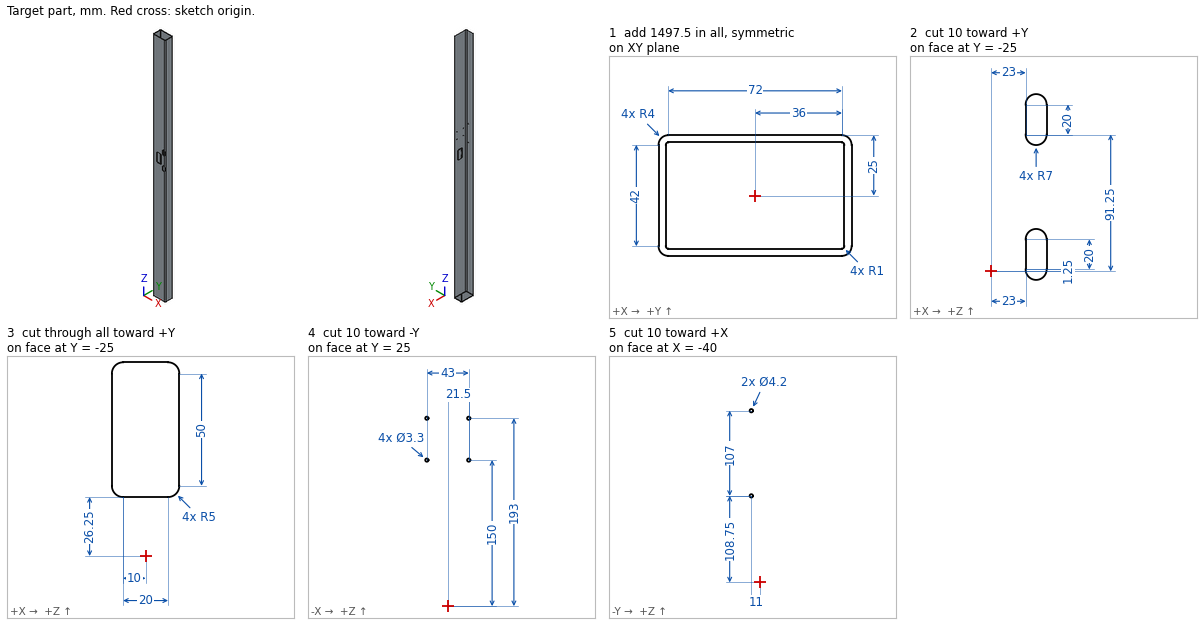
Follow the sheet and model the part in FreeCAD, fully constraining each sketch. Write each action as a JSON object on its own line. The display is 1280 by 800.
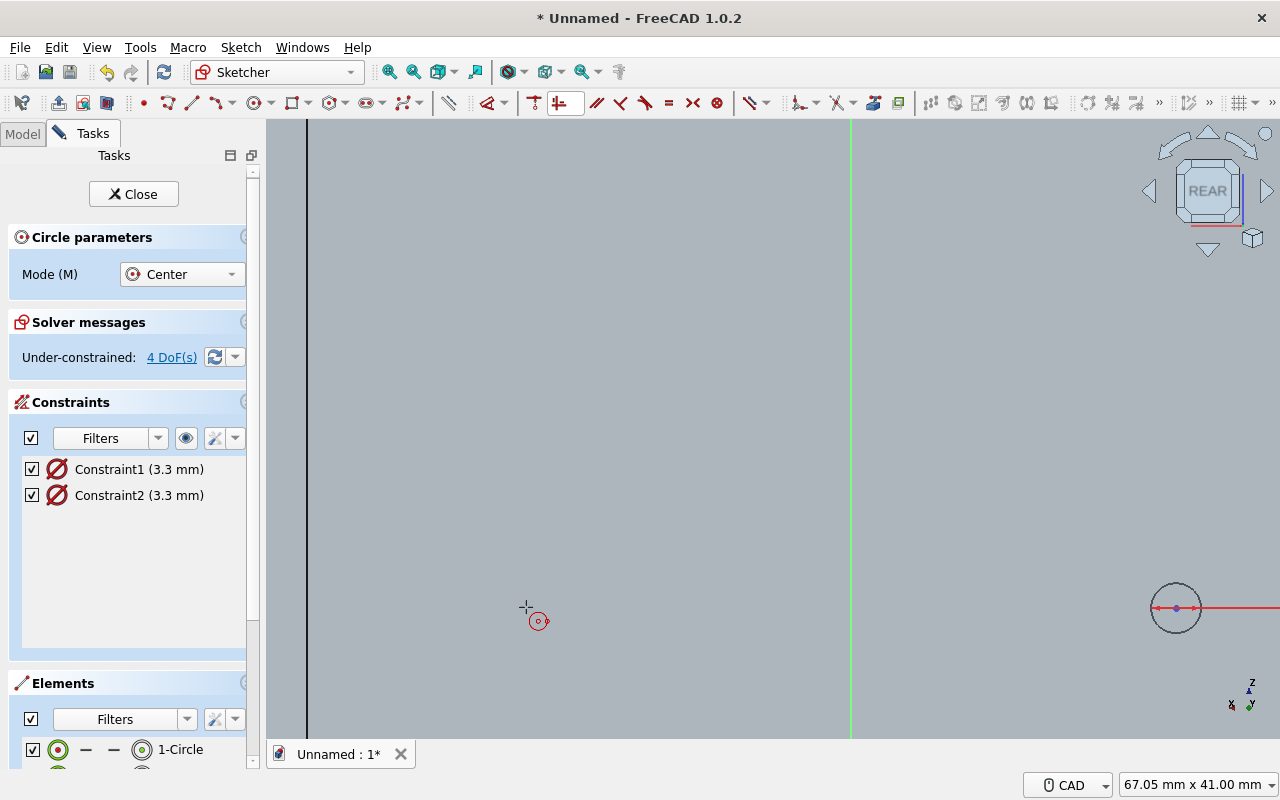
{"action": "left_click", "coordinate": [526, 607]}
{"action": "mouse_move", "coordinate": [544, 589]}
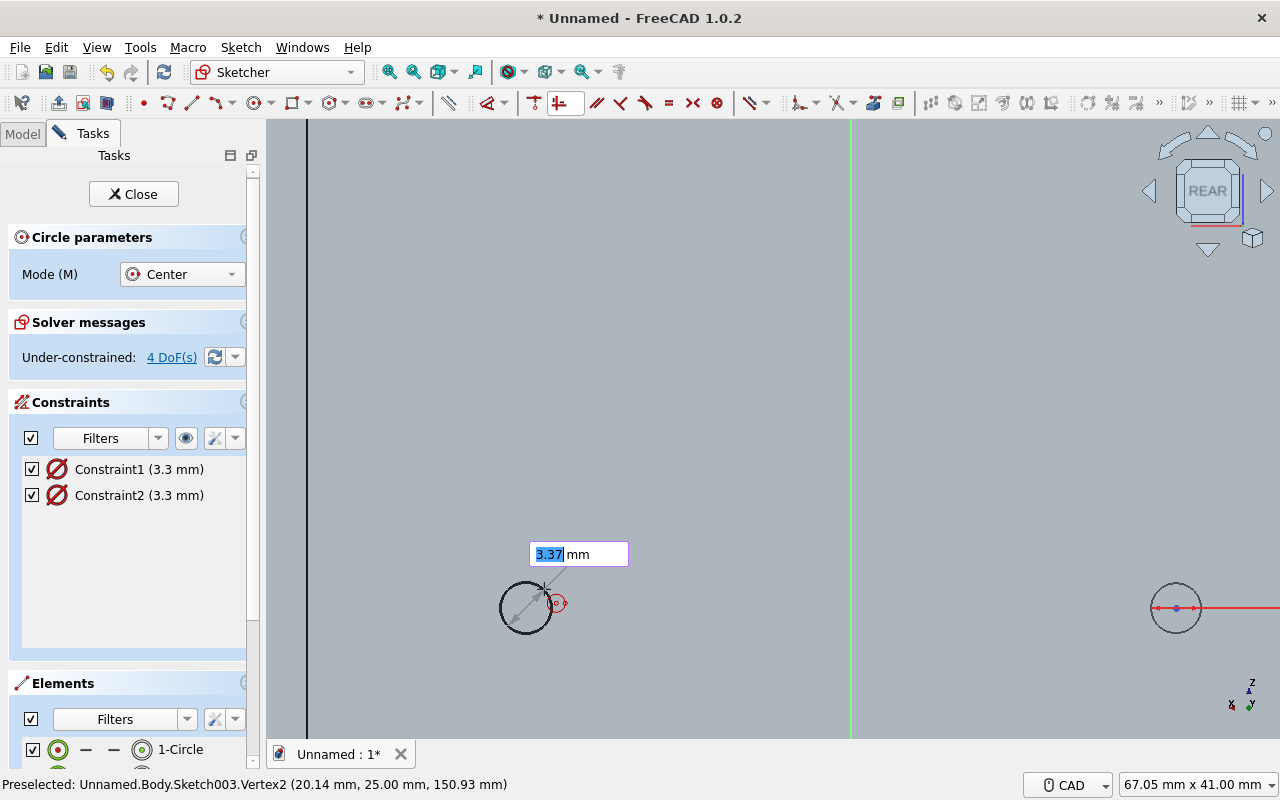
{"action": "type", "text": "3.3"}
{"action": "key", "text": "Return"}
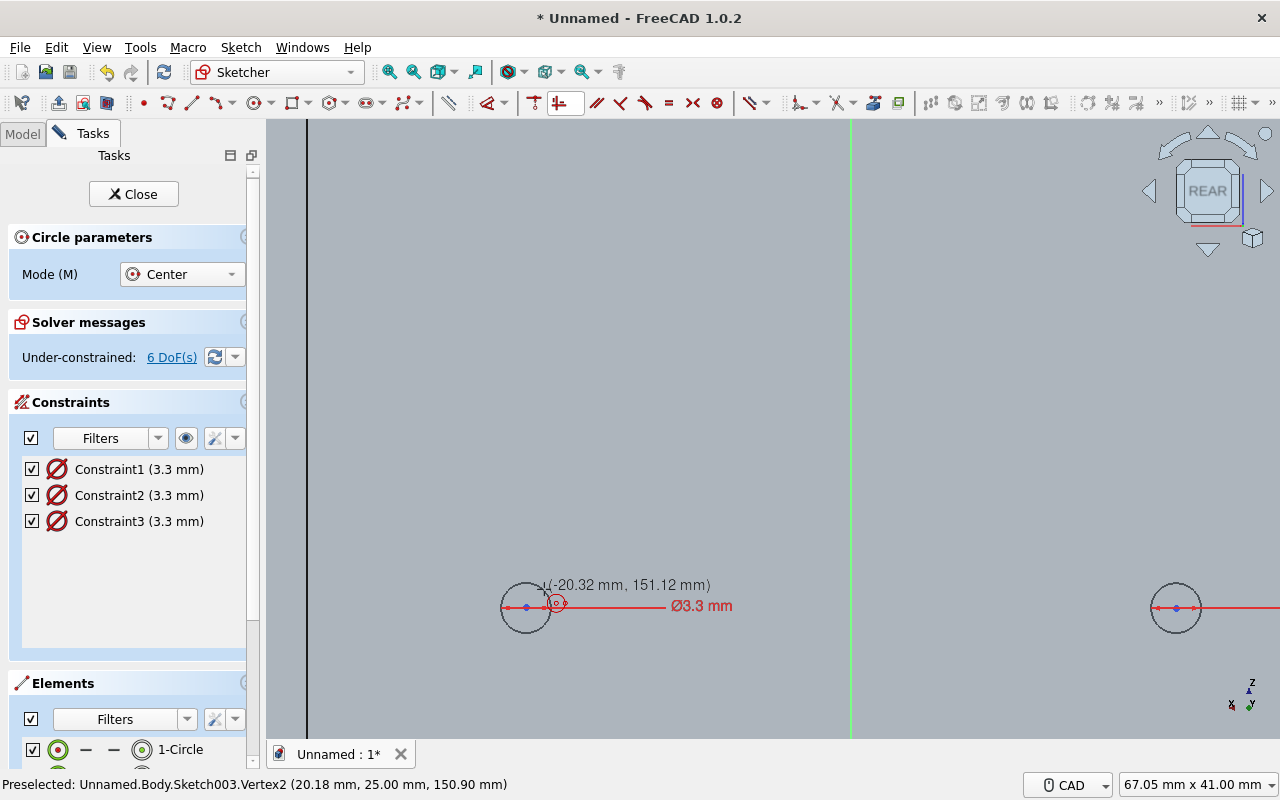
{"action": "scroll", "coordinate": [526, 608], "scroll_direction": "down", "scroll_amount": 3}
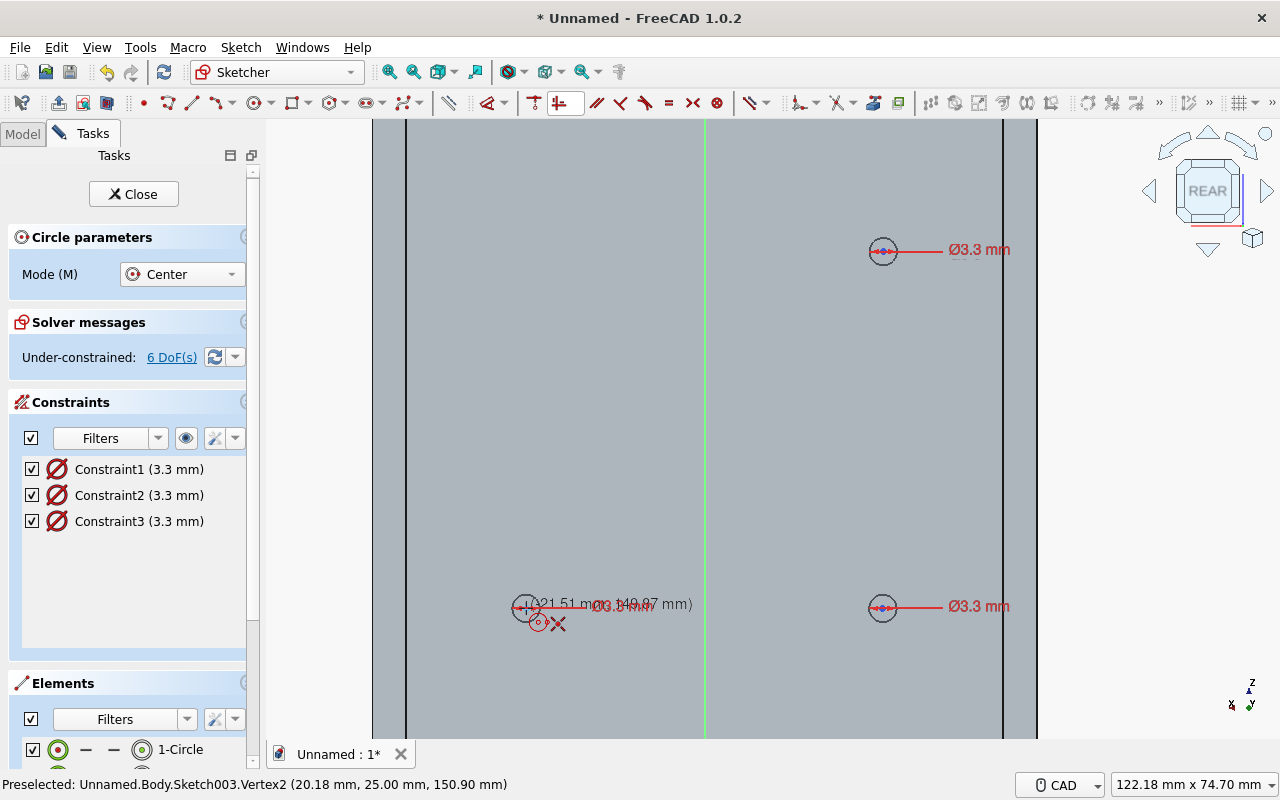
{"action": "scroll", "coordinate": [526, 251], "scroll_direction": "up", "scroll_amount": 3}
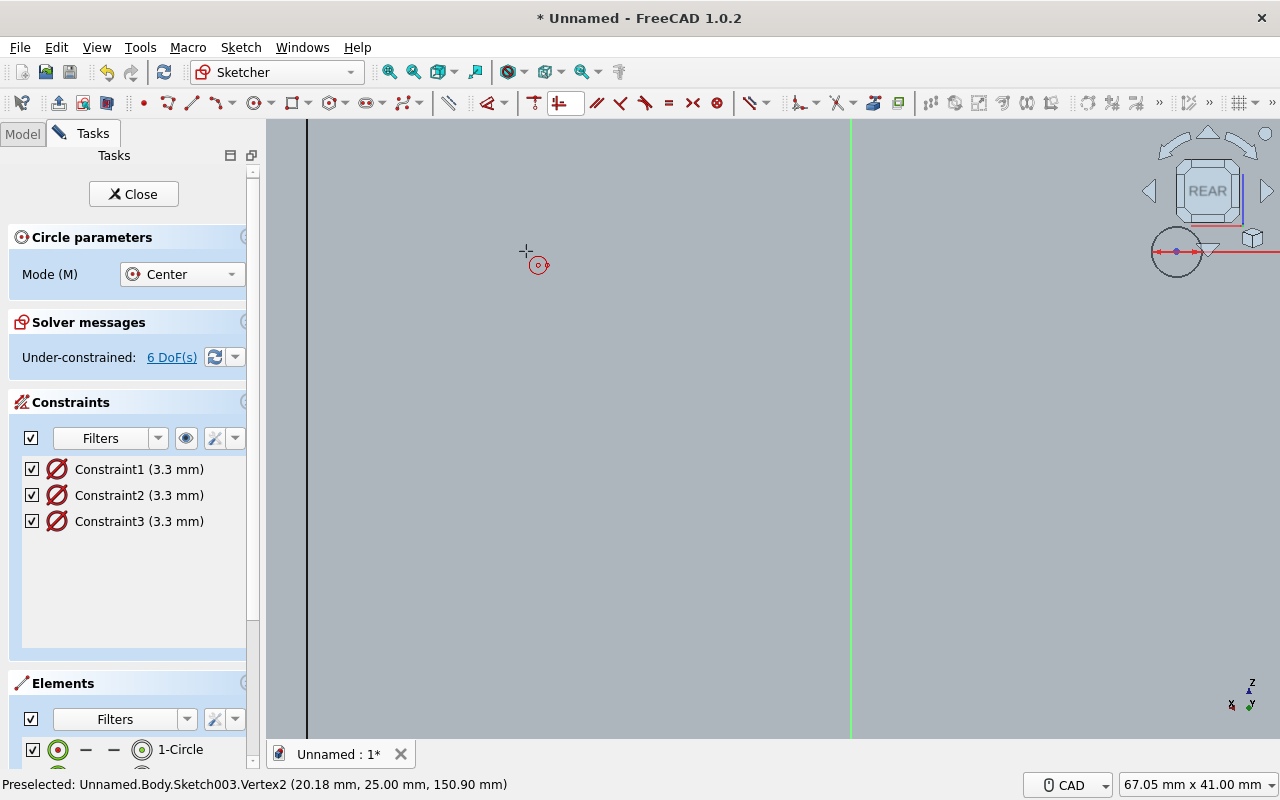
{"action": "left_click", "coordinate": [526, 251]}
{"action": "mouse_move", "coordinate": [544, 233]}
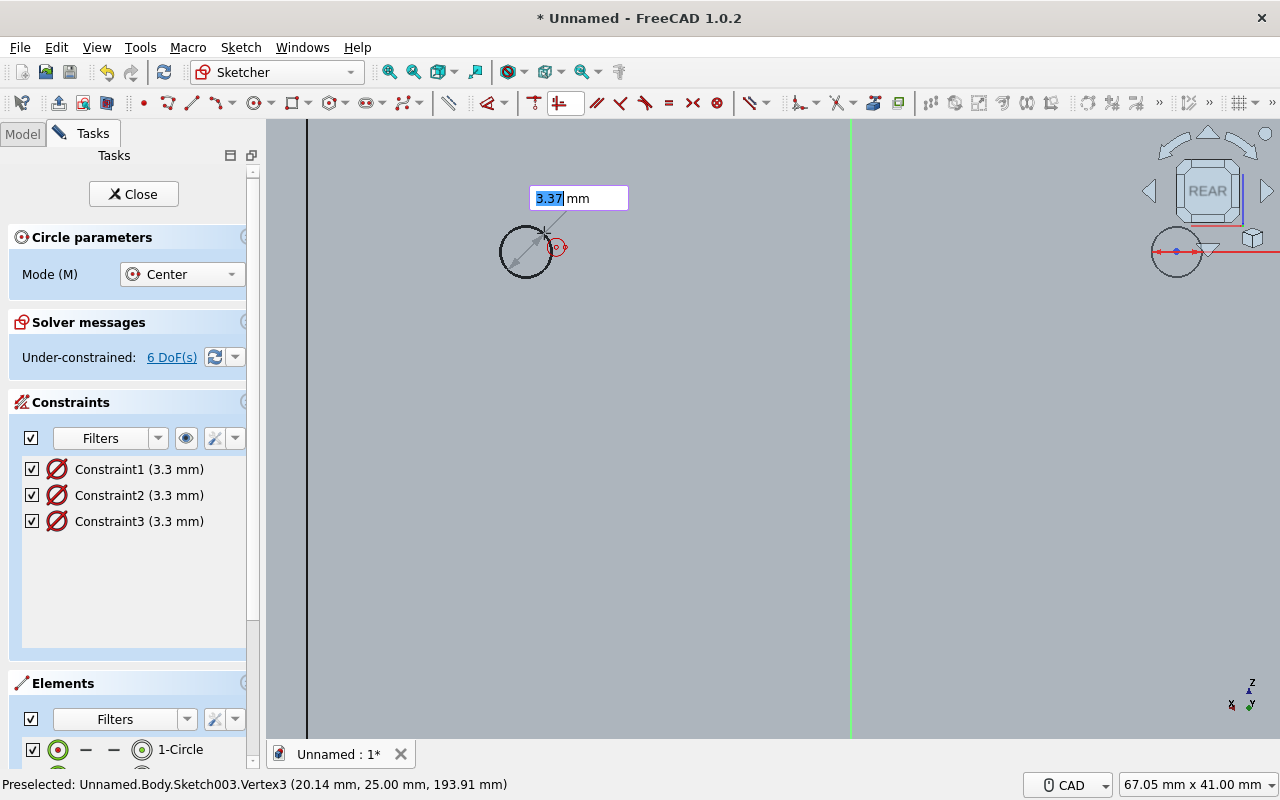
{"action": "type", "text": "3.3"}
{"action": "key", "text": "Return"}
{"action": "key", "text": "Escape"}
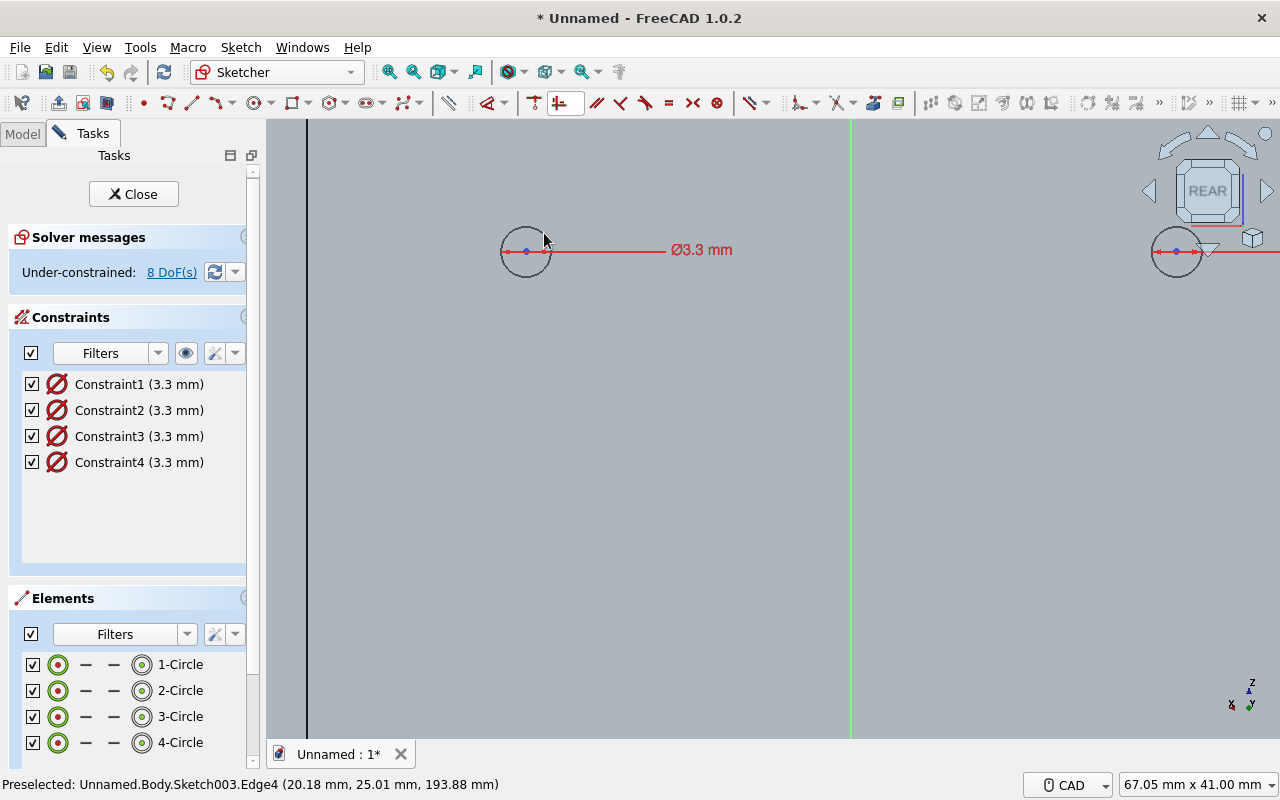
{"action": "scroll", "coordinate": [526, 250], "scroll_direction": "down", "scroll_amount": 3}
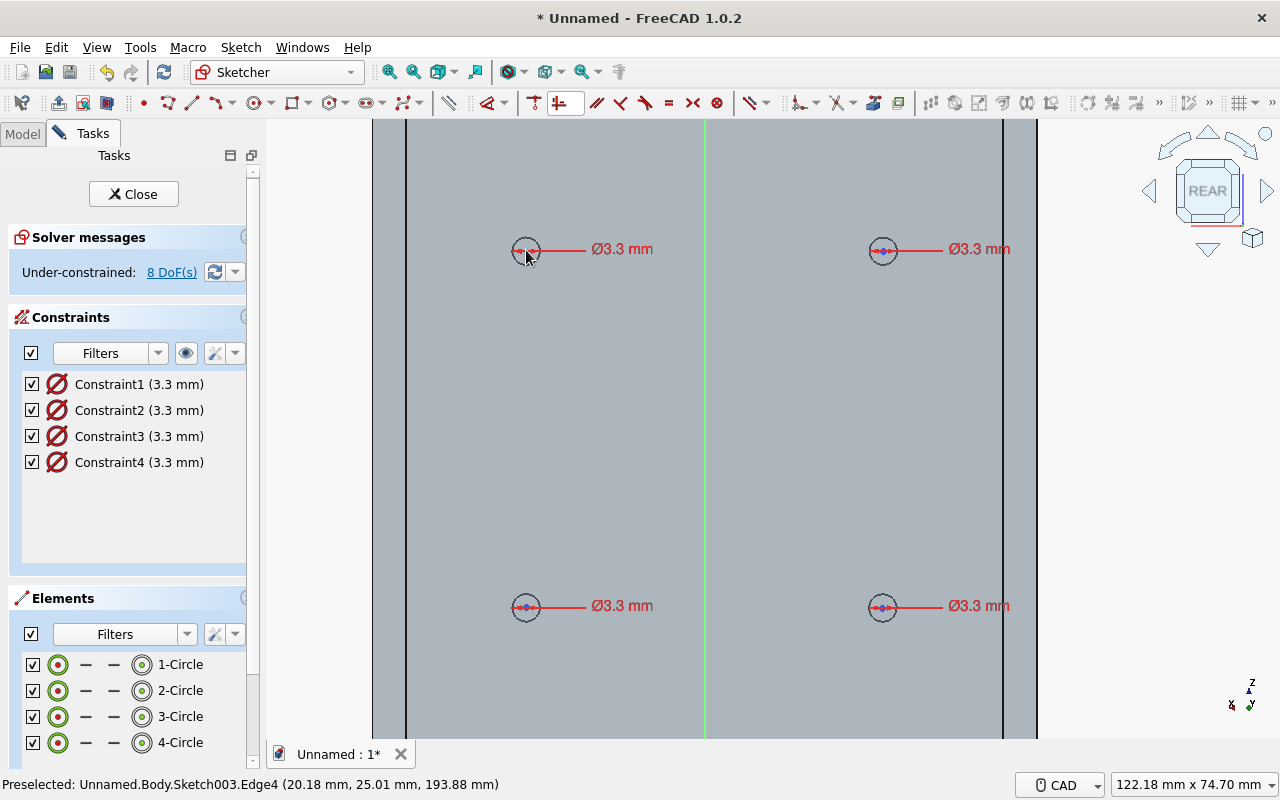
{"action": "left_click", "coordinate": [883, 608]}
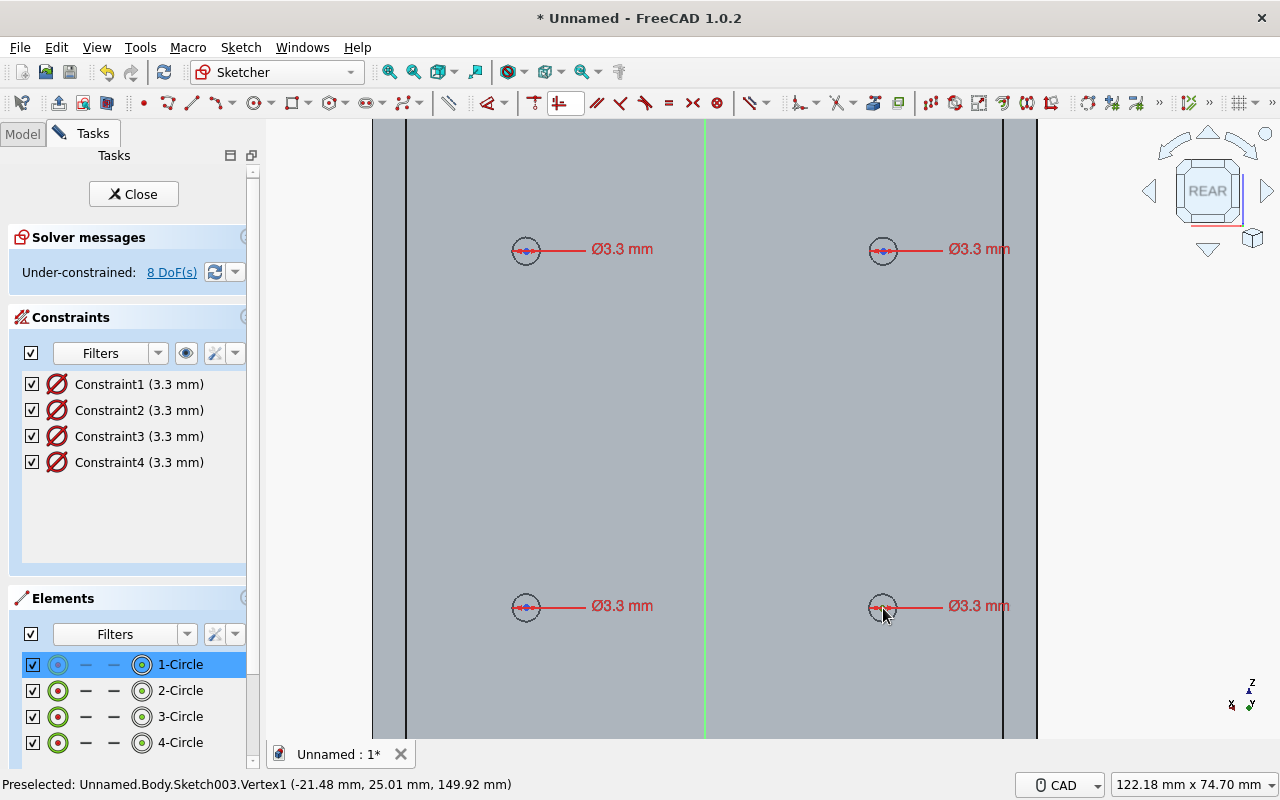
{"action": "left_click", "coordinate": [883, 251]}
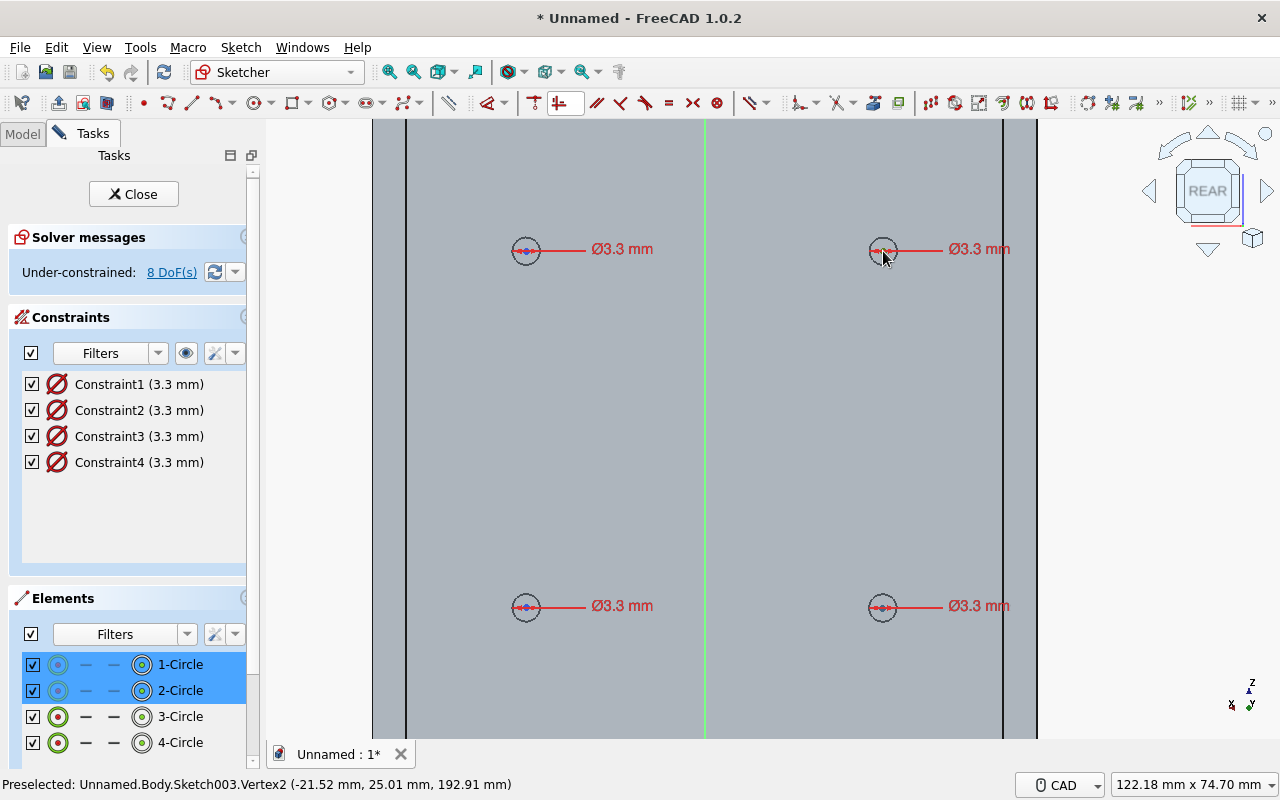
{"action": "key", "text": "v"}